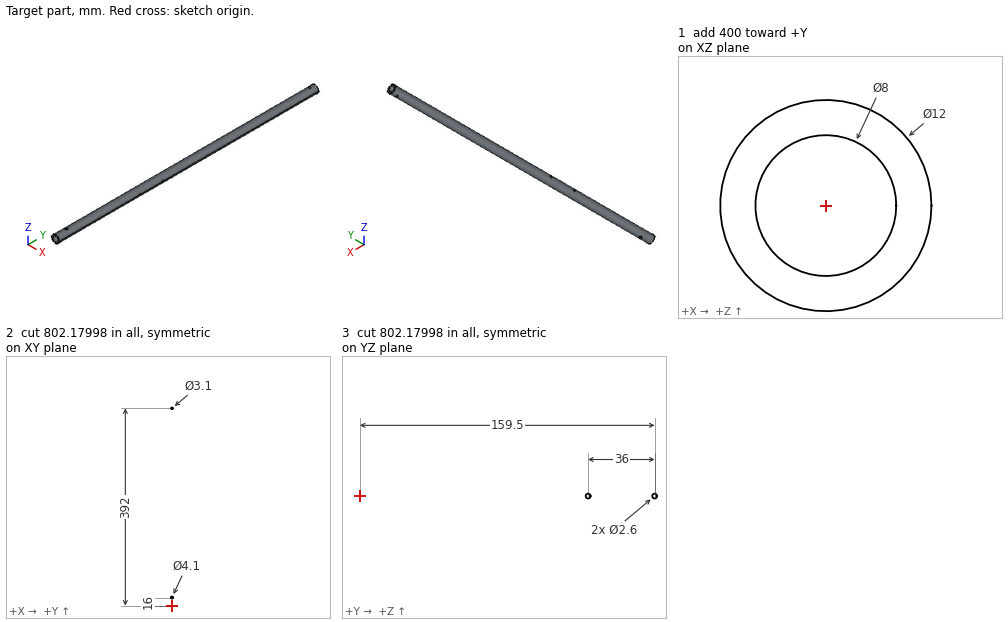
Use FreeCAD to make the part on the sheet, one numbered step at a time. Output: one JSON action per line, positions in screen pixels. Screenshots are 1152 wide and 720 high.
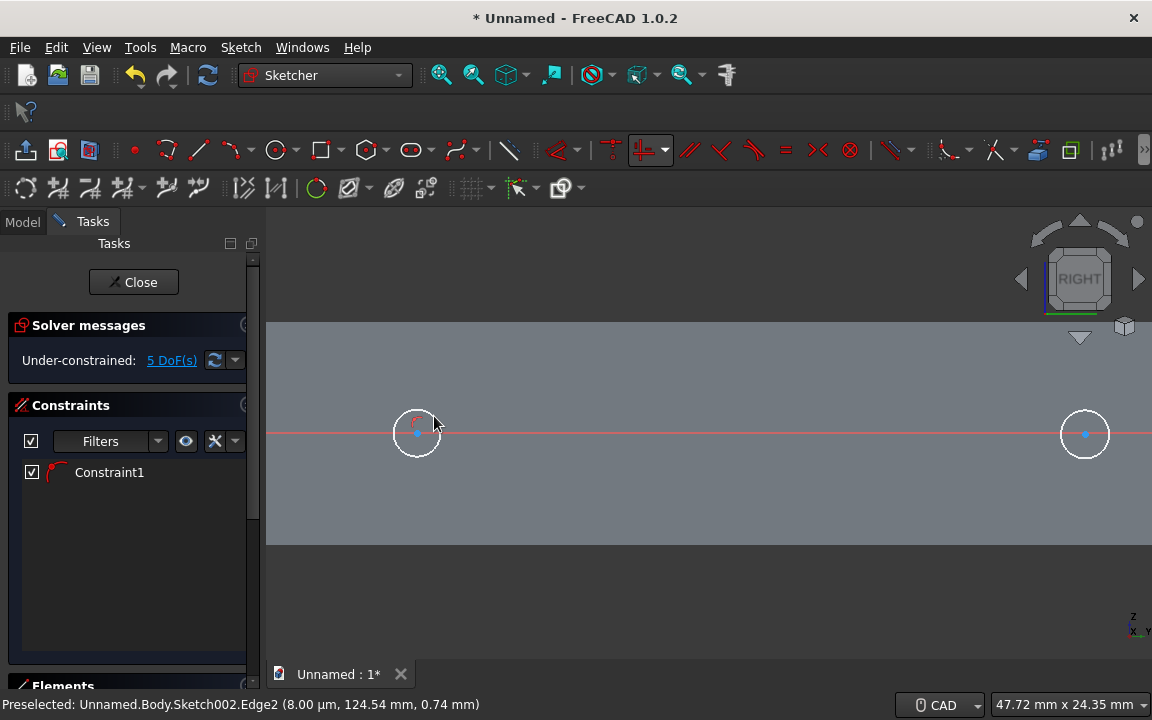
{"action": "scroll", "coordinate": [416, 433], "scroll_direction": "down", "scroll_amount": 2}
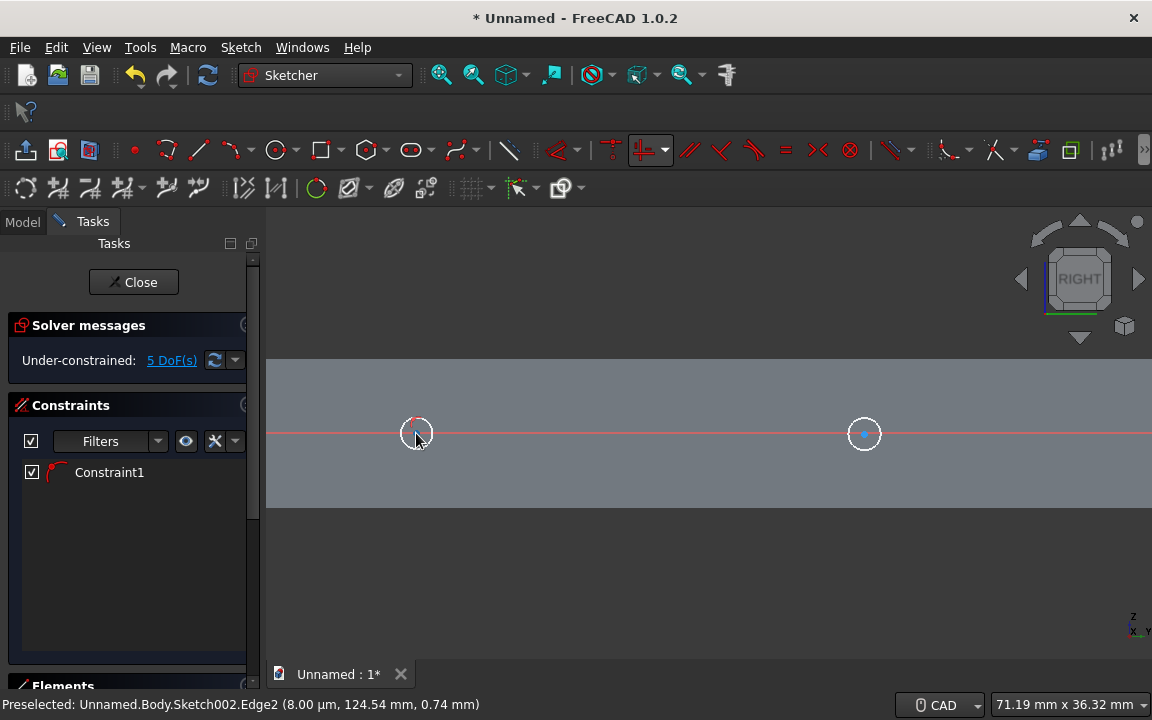
{"action": "scroll", "coordinate": [876, 423], "scroll_direction": "up", "scroll_amount": 2}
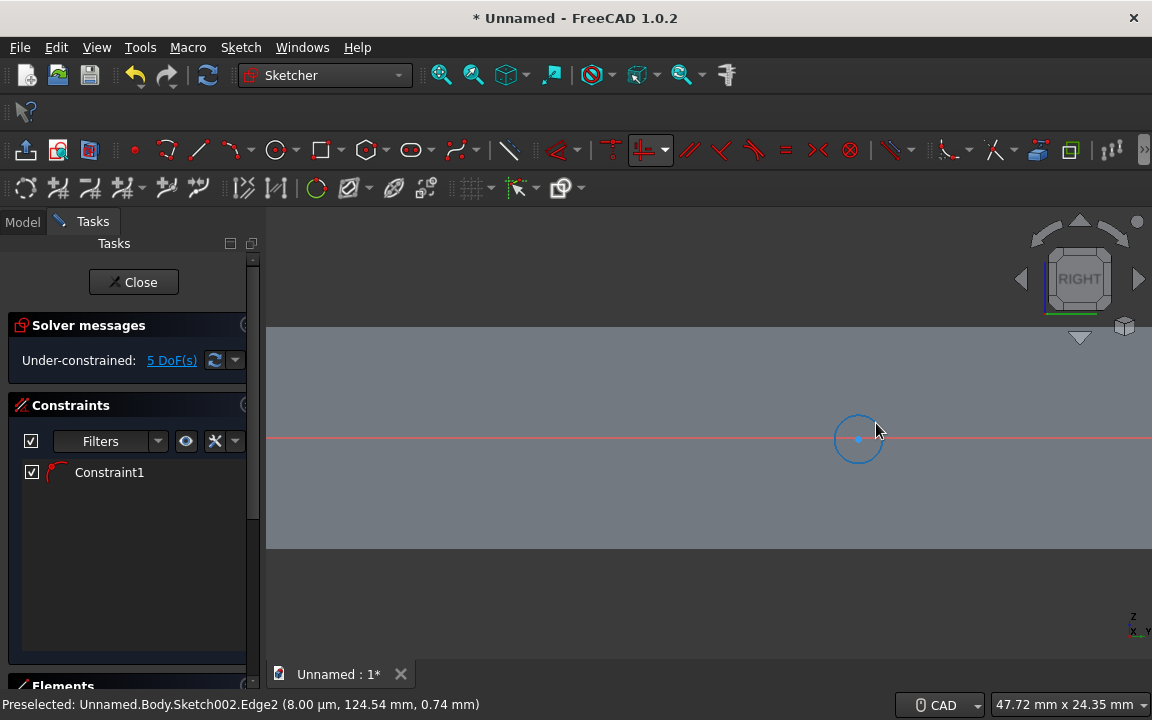
{"action": "left_click", "coordinate": [876, 422]}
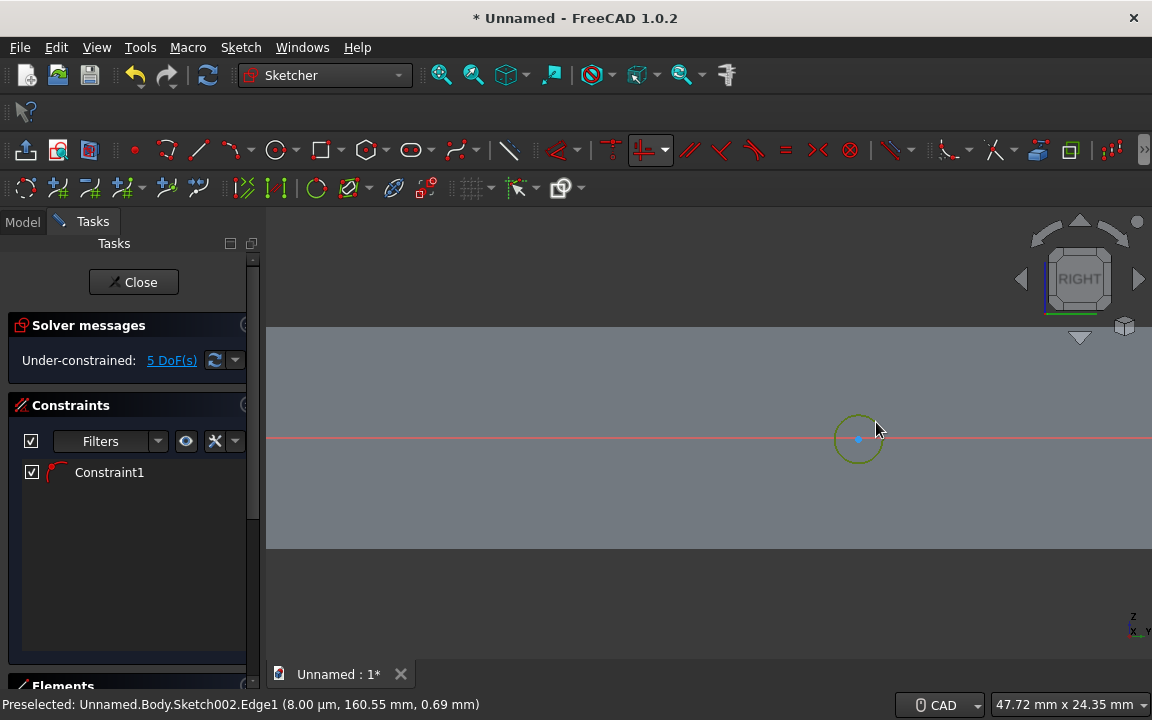
{"action": "scroll", "coordinate": [877, 423], "scroll_direction": "down", "scroll_amount": 2}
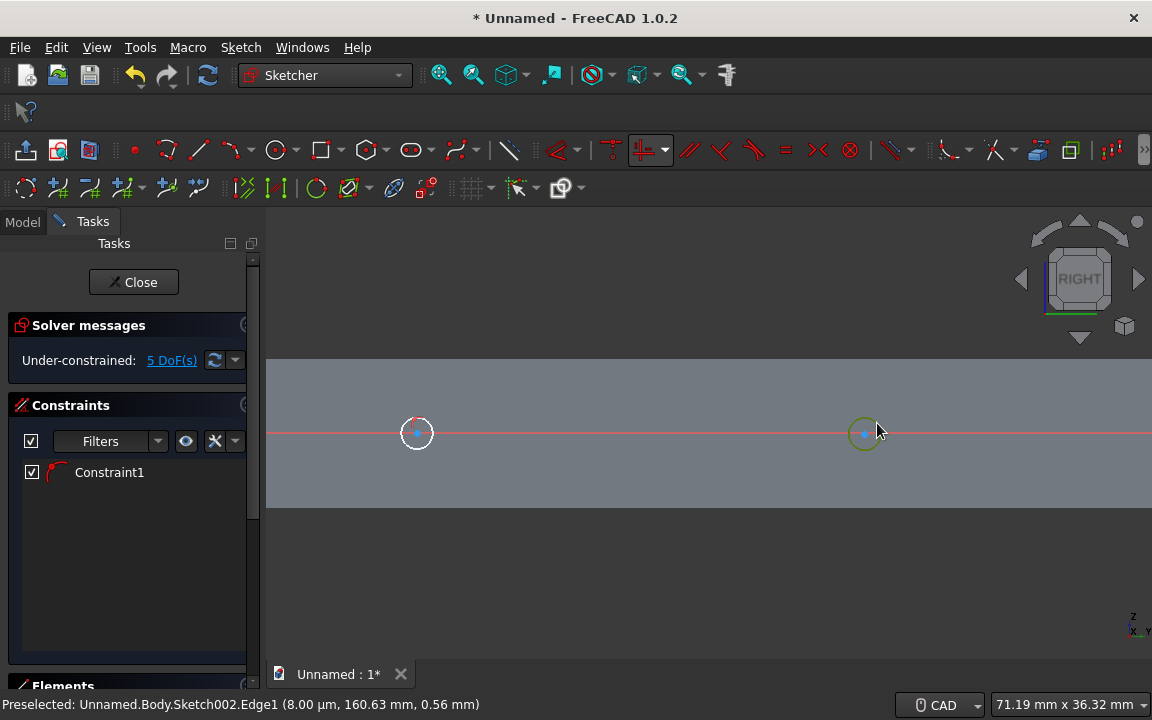
{"action": "scroll", "coordinate": [428, 422], "scroll_direction": "up", "scroll_amount": 2}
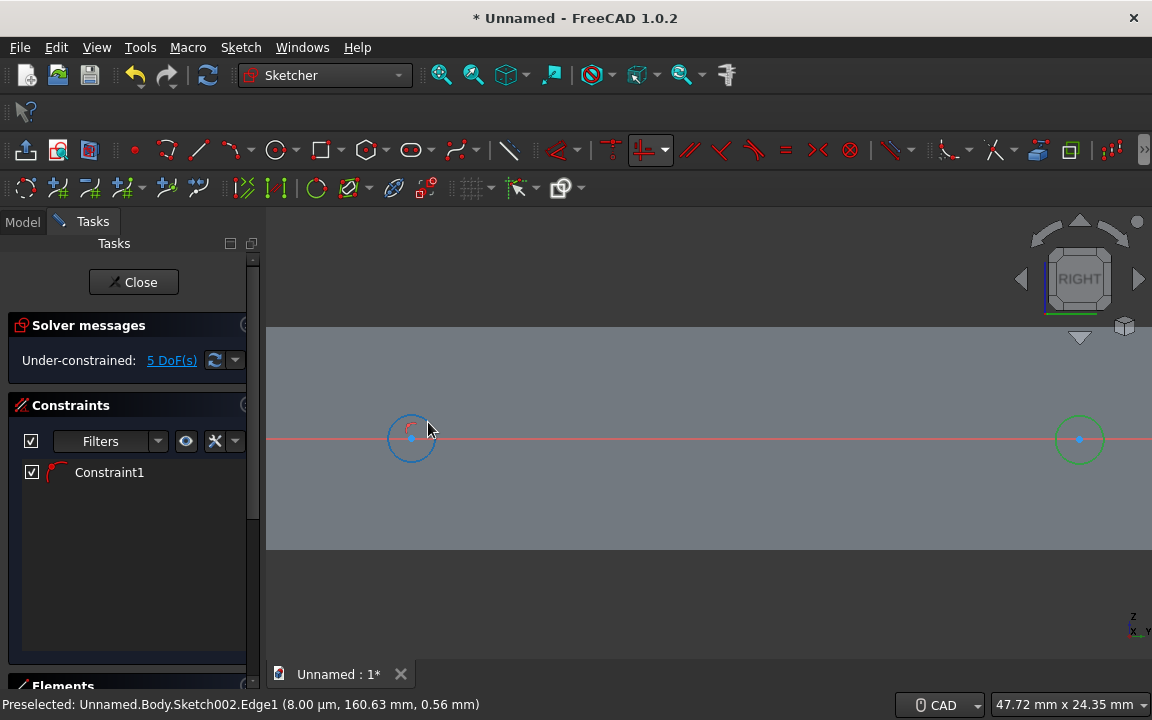
{"action": "left_click", "coordinate": [428, 422]}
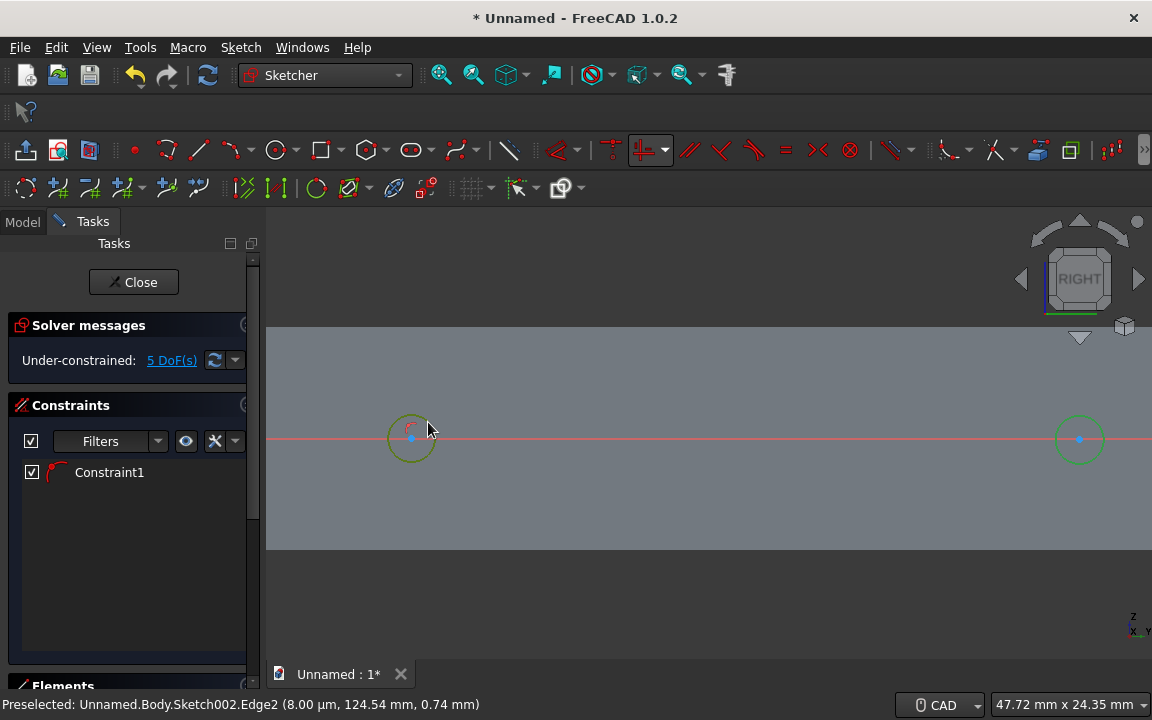
{"action": "key", "text": "e"}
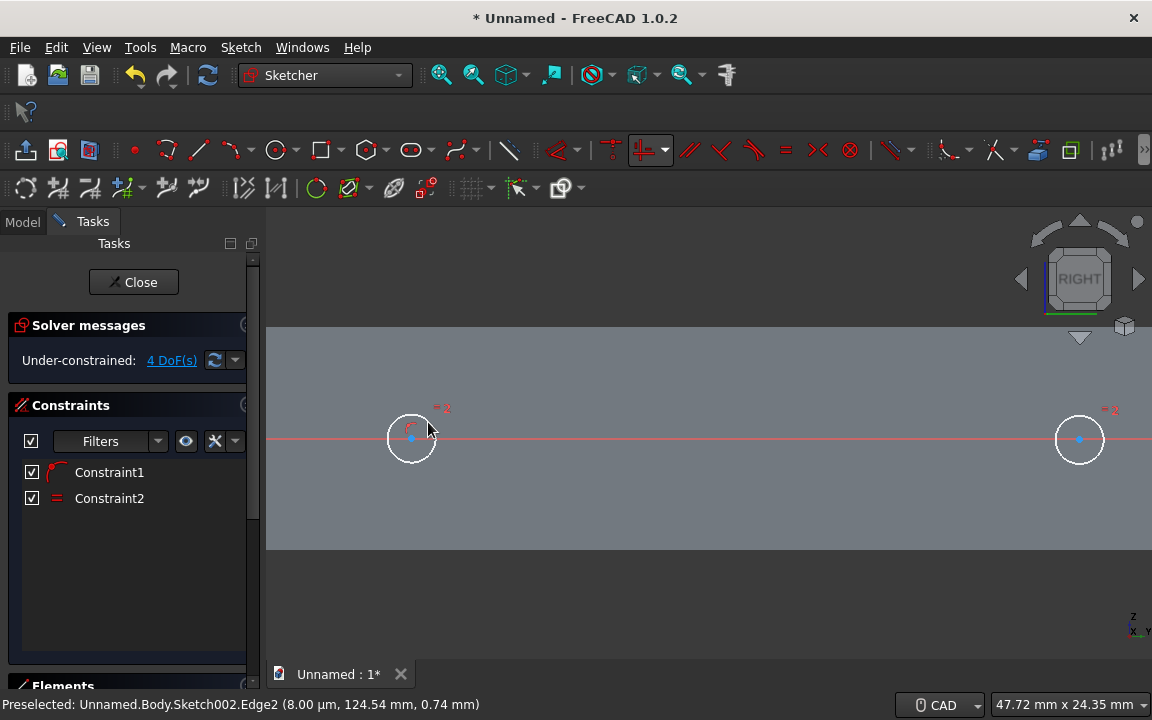
{"action": "scroll", "coordinate": [427, 422], "scroll_direction": "down", "scroll_amount": 2}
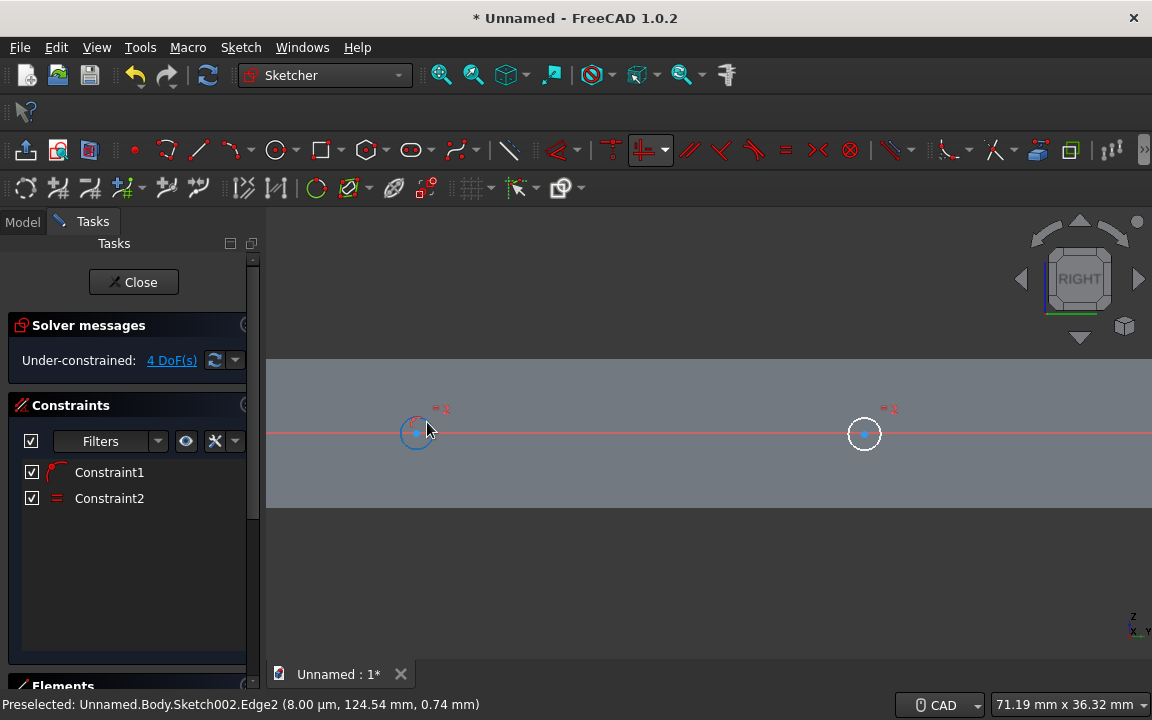
{"action": "left_click", "coordinate": [865, 434]}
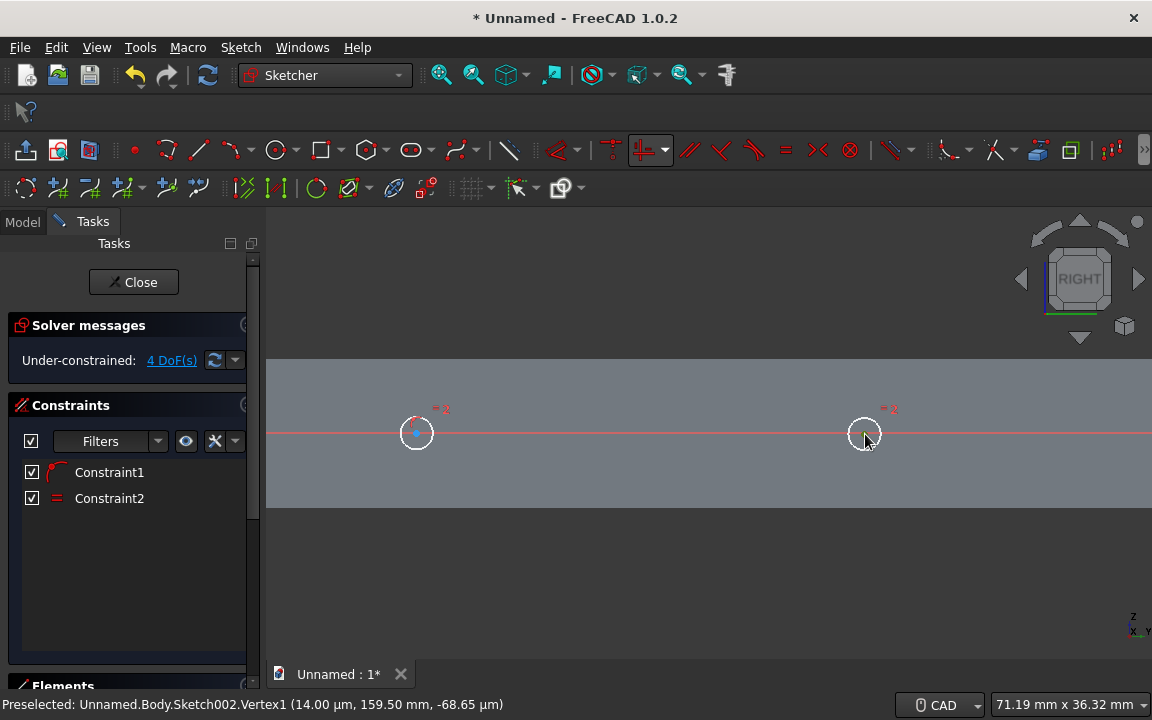
{"action": "left_click", "coordinate": [344, 433]}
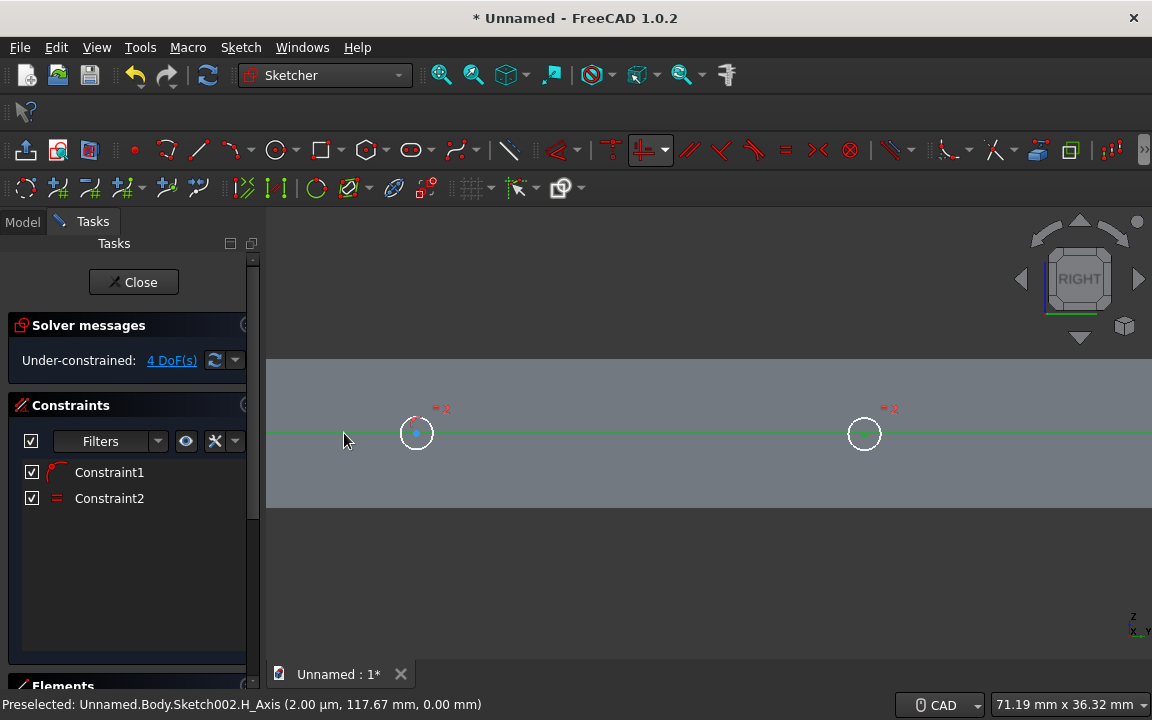
{"action": "key", "text": "c"}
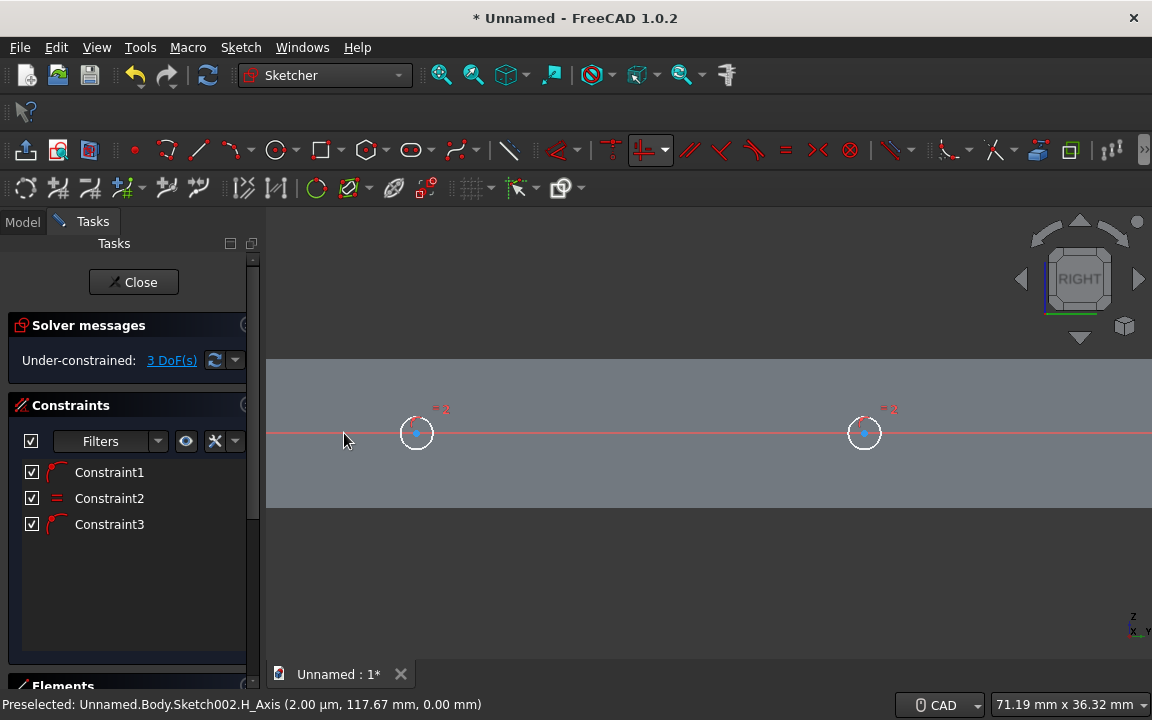
{"action": "key", "text": "d"}